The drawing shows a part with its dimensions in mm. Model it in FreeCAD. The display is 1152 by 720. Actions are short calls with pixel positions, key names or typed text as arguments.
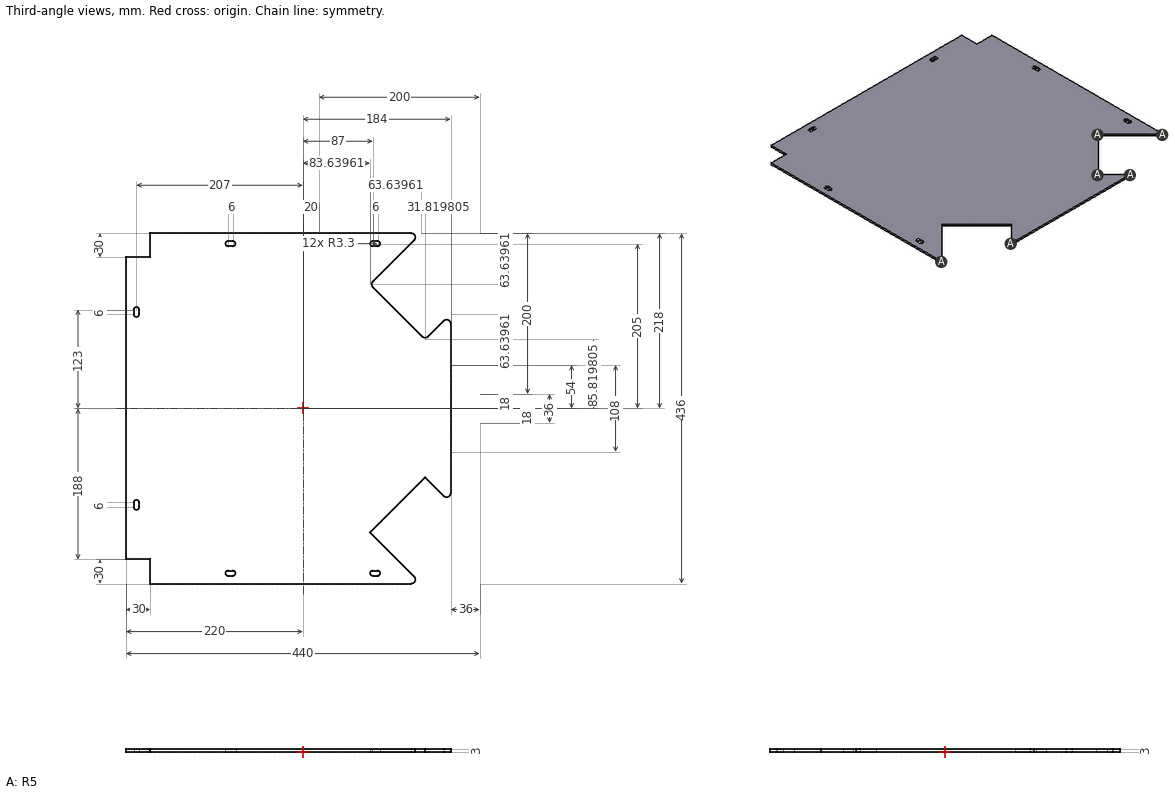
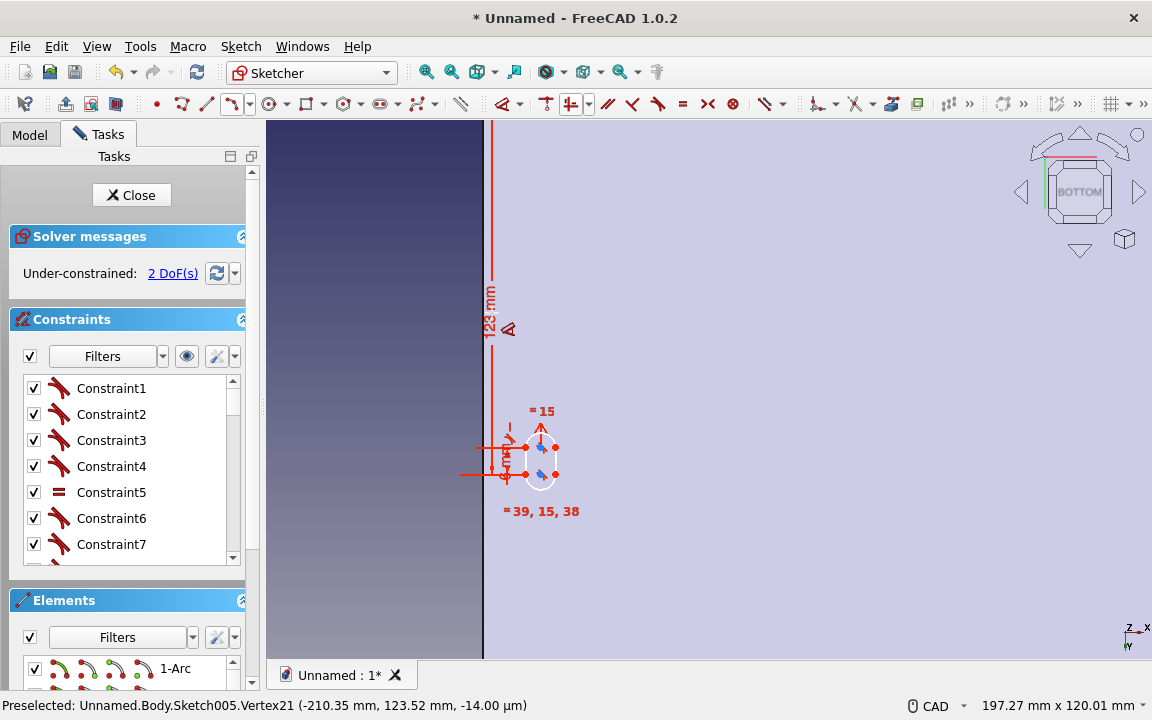
scroll(527, 482, down, 9)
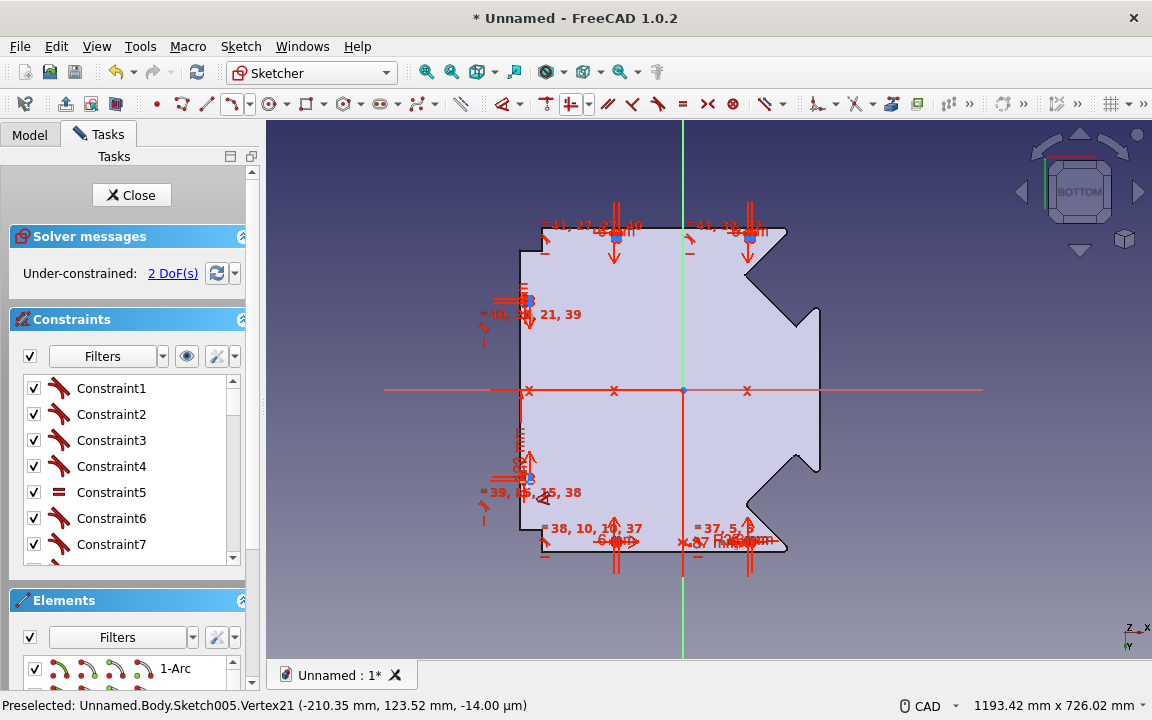
scroll(748, 542, up, 9)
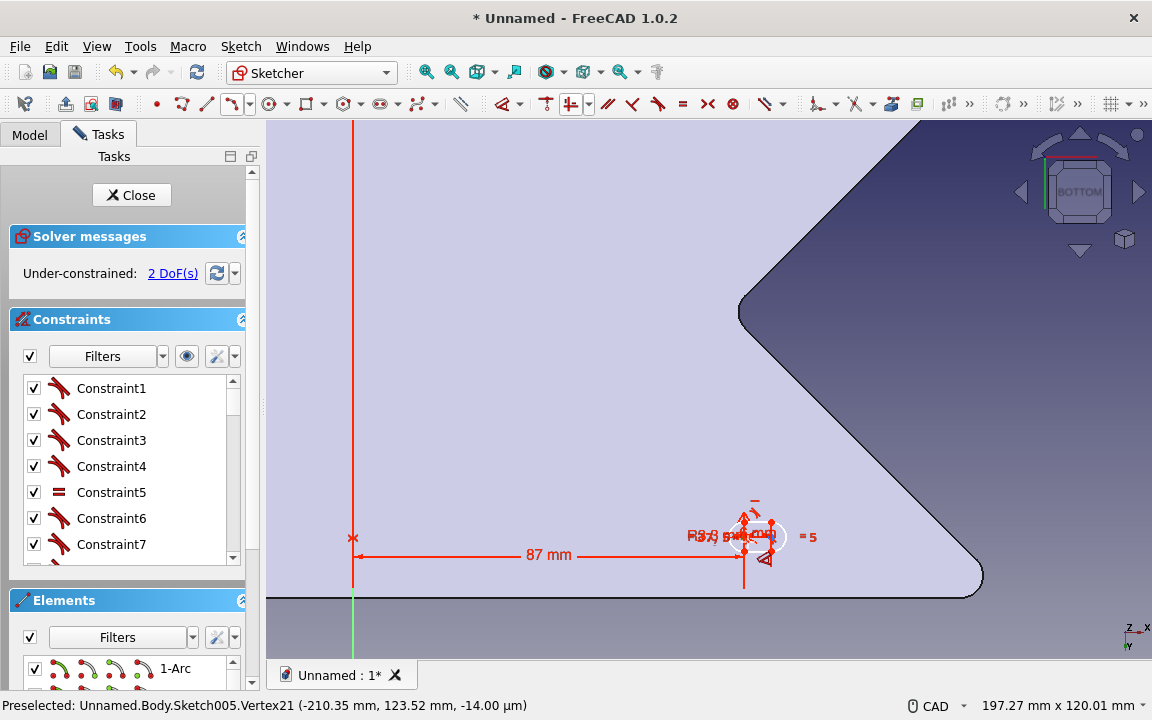
click(744, 537)
click(778, 343)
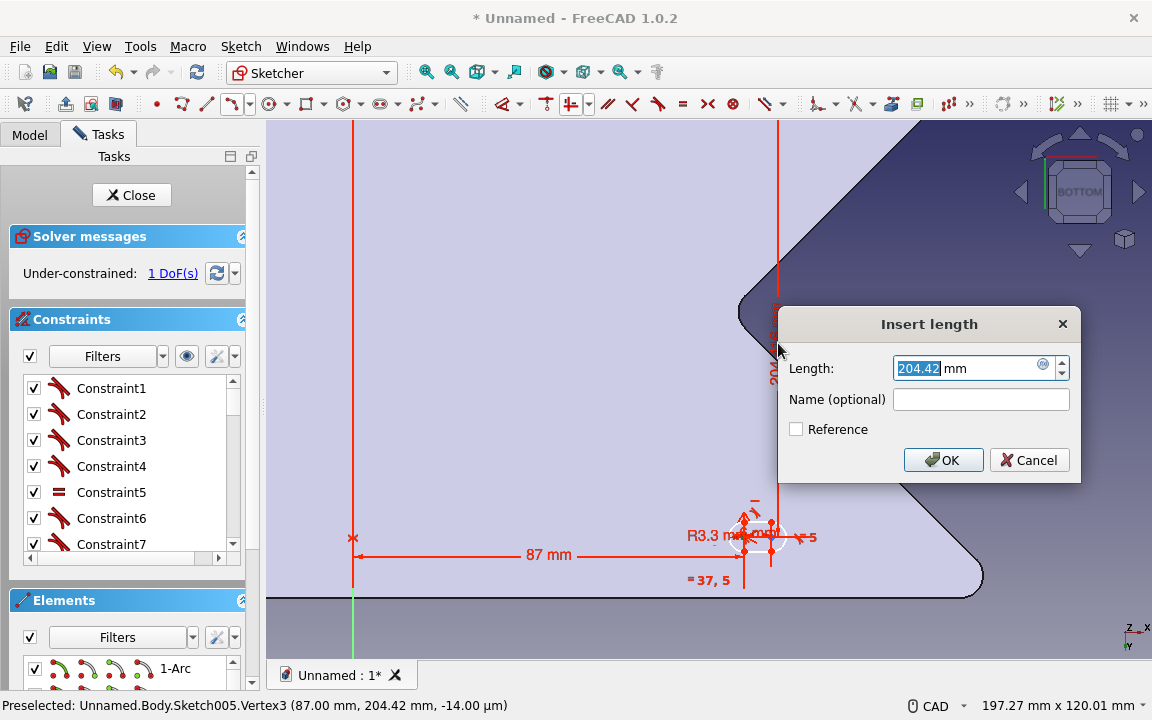
text(205)
key(Return)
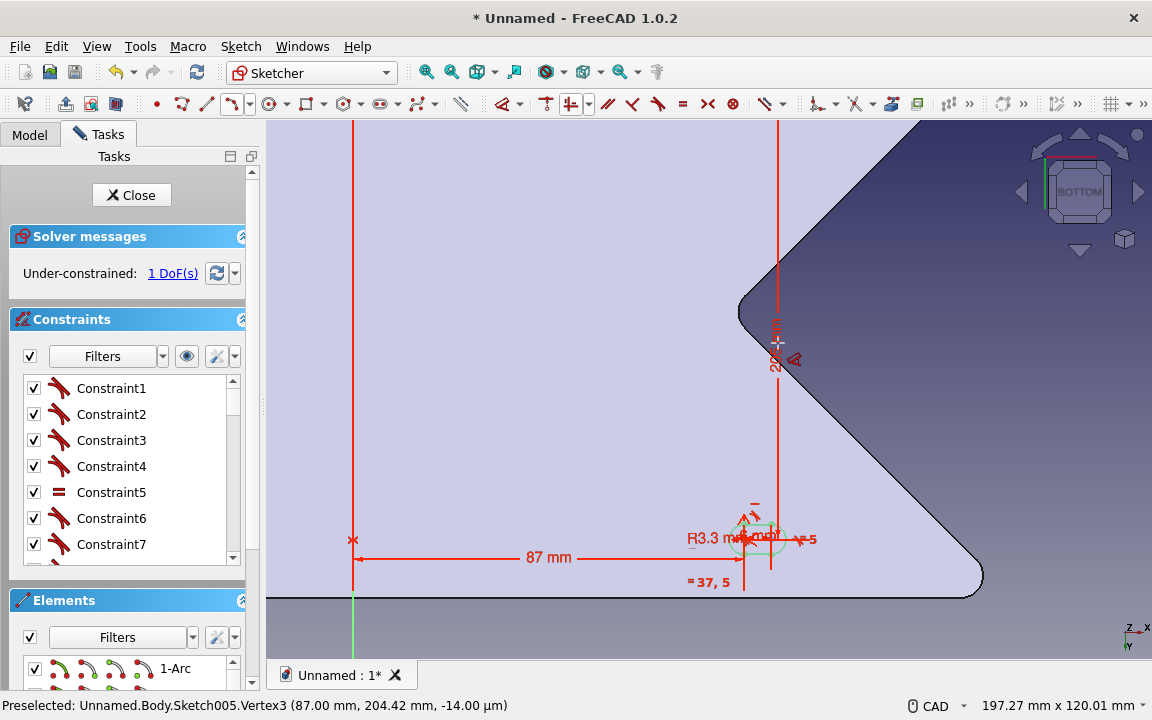
scroll(748, 542, down, 9)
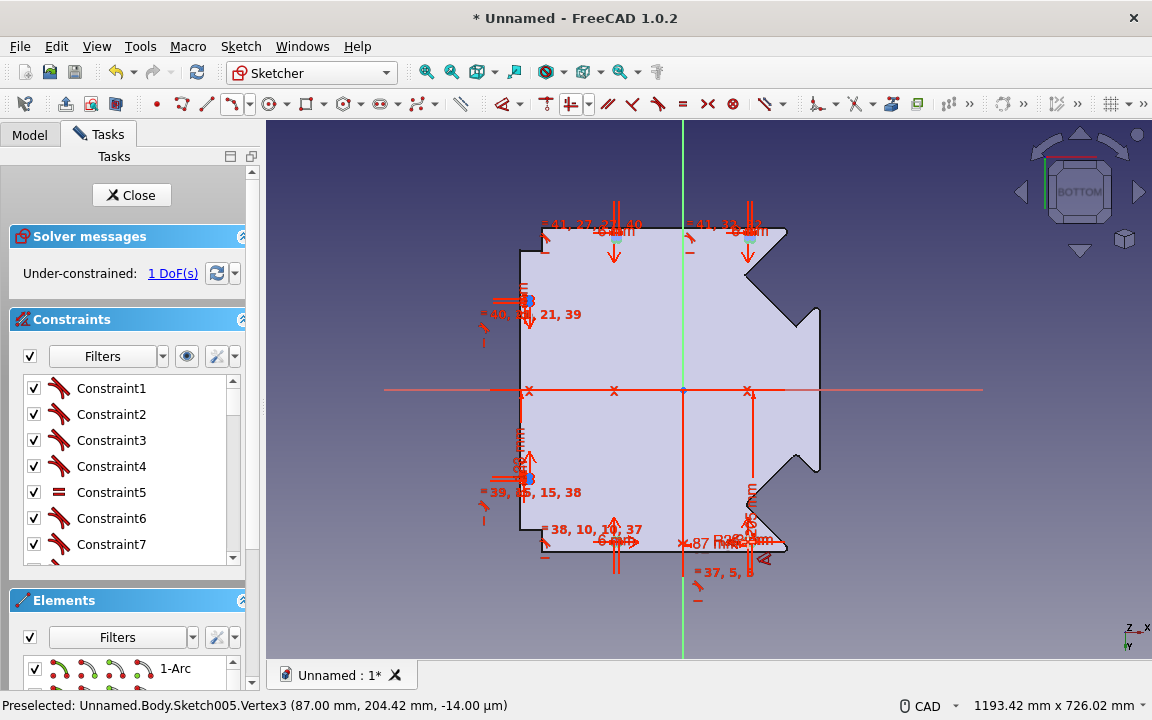
scroll(530, 481, up, 9)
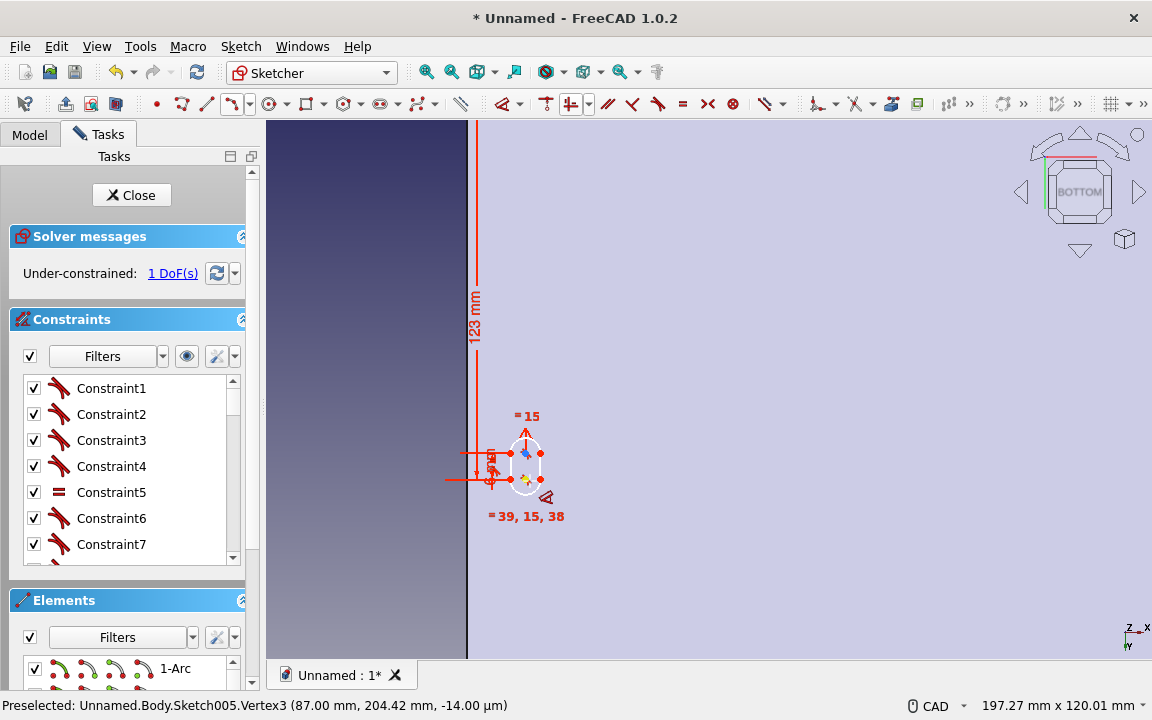
click(526, 480)
click(756, 514)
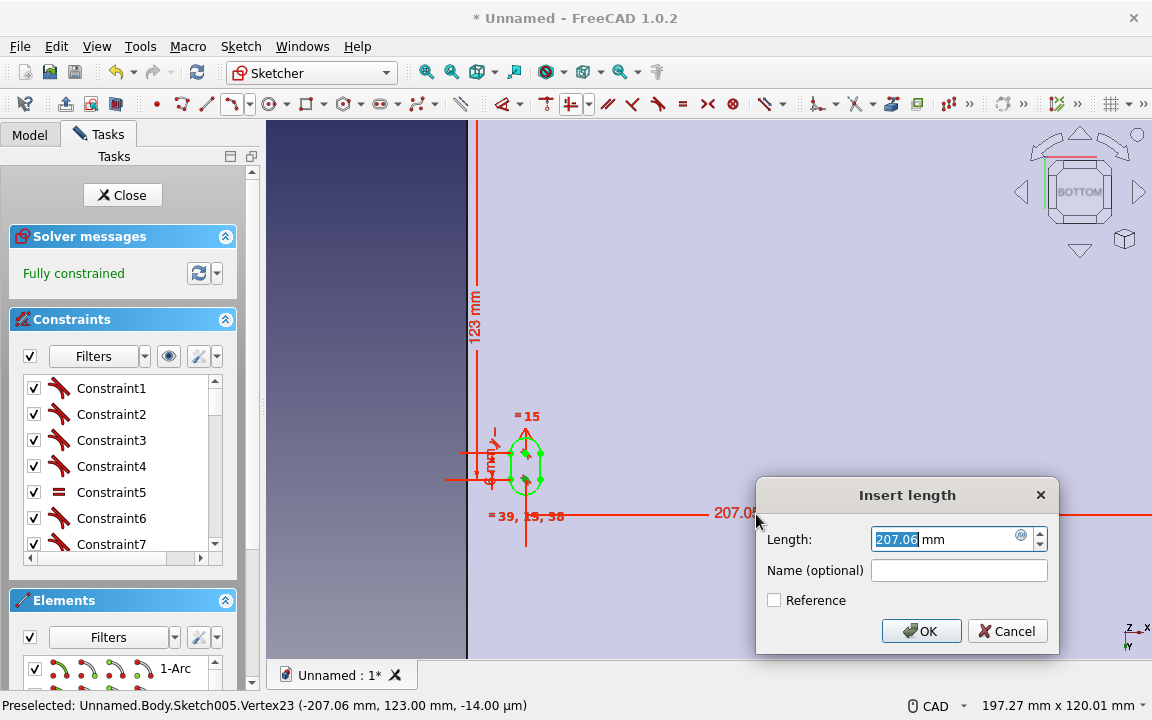
text(207)
key(Return)
key(Escape)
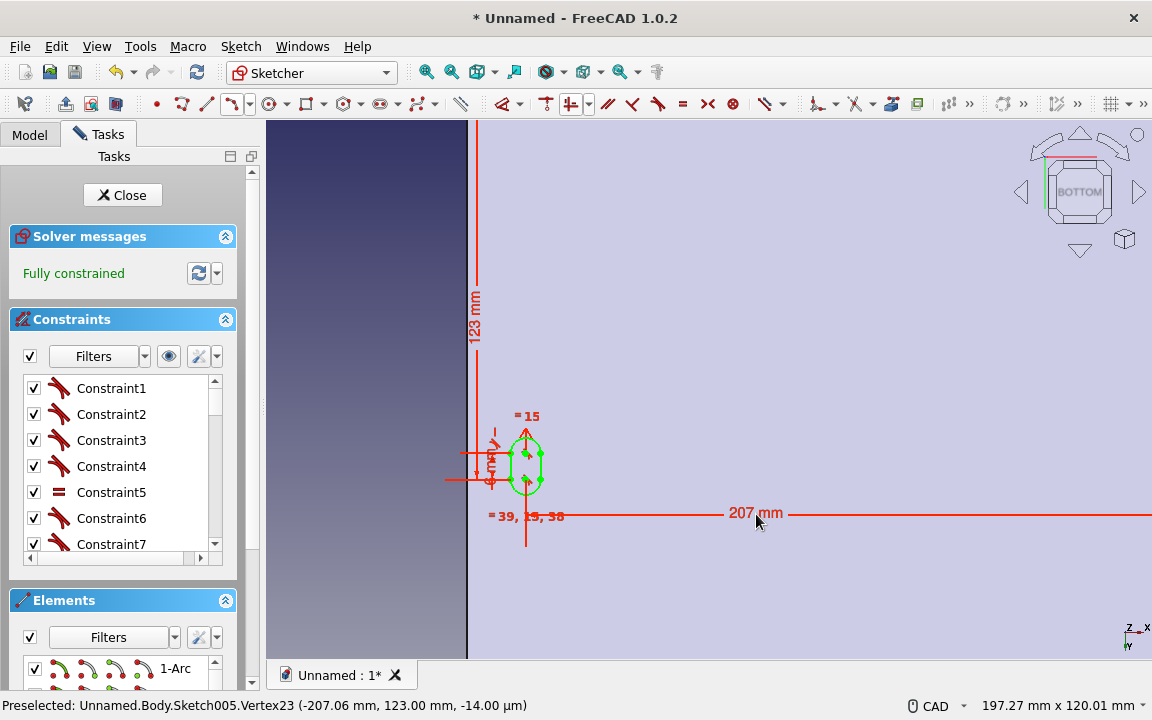
click(123, 195)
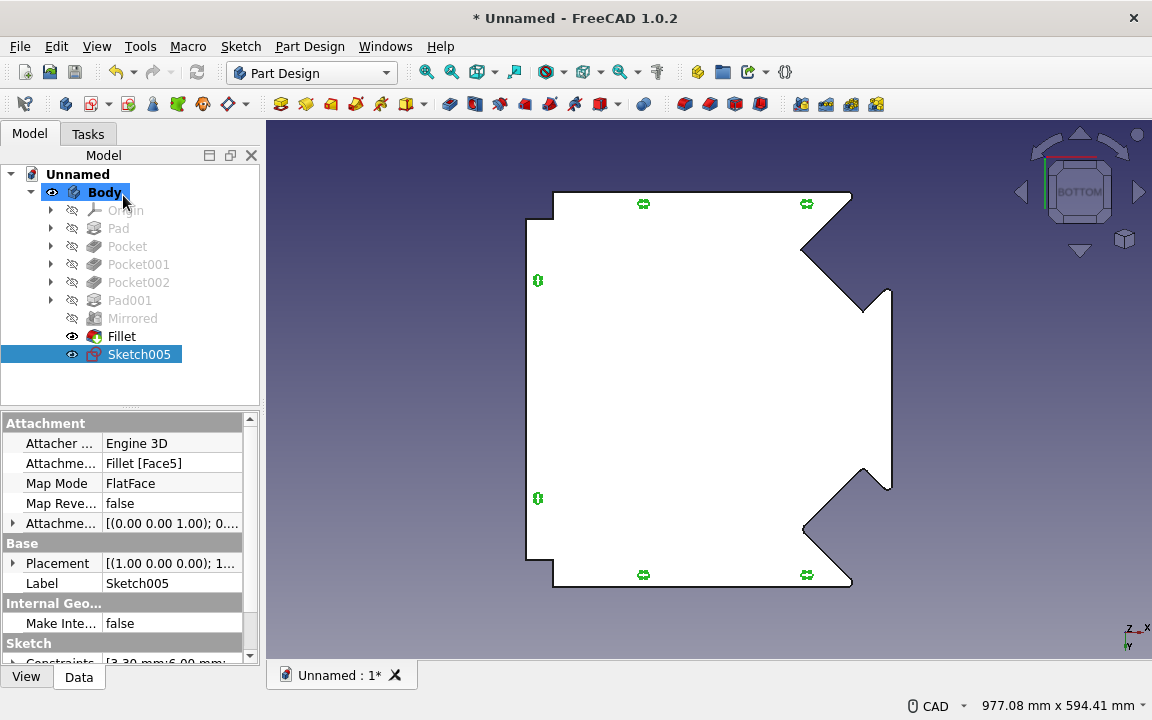
click(450, 104)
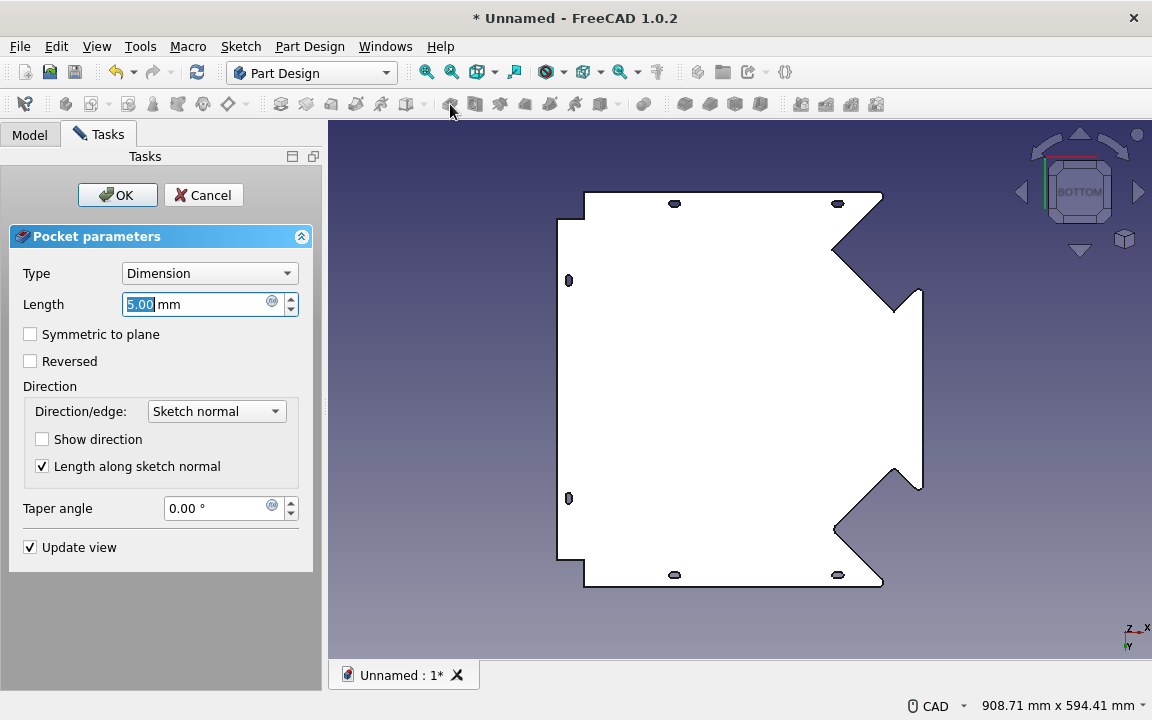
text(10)
key(Tab)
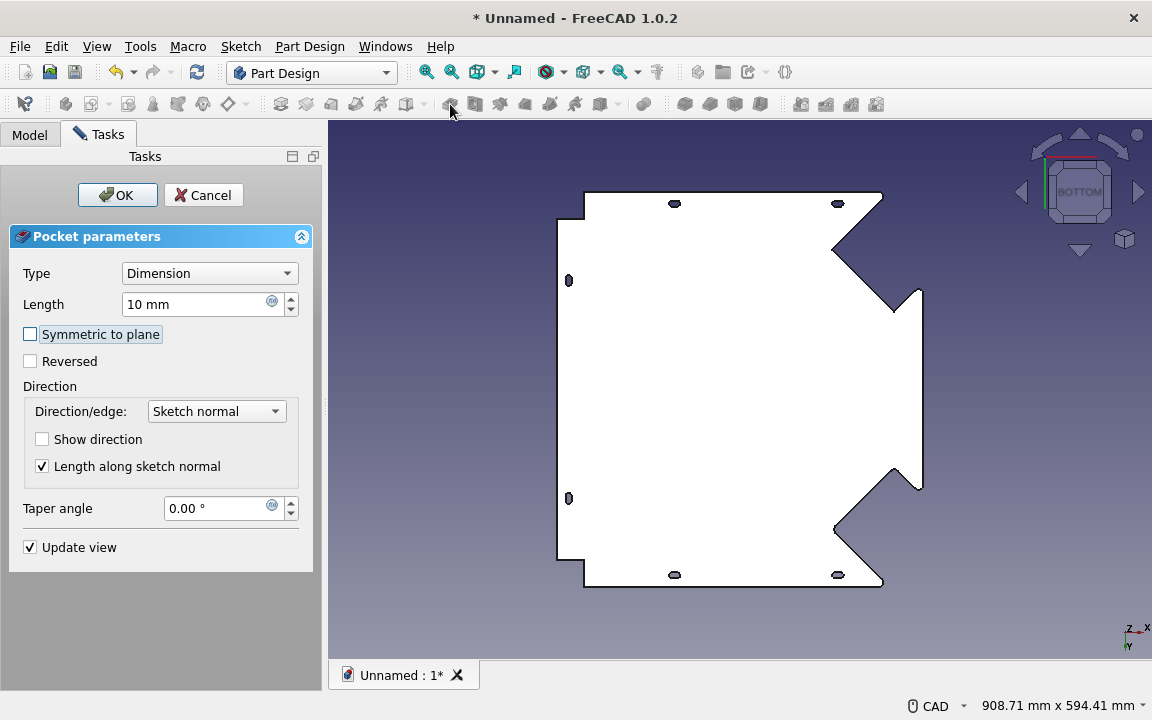
click(118, 195)